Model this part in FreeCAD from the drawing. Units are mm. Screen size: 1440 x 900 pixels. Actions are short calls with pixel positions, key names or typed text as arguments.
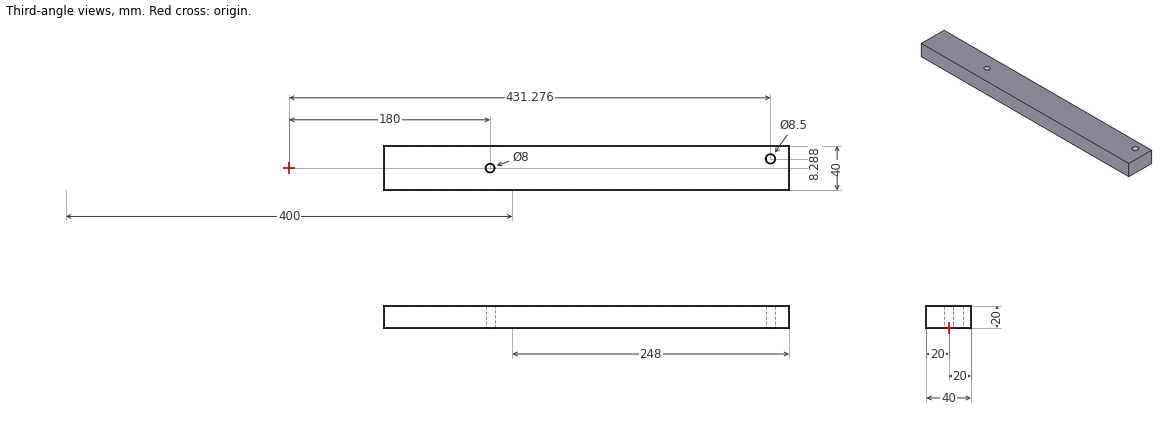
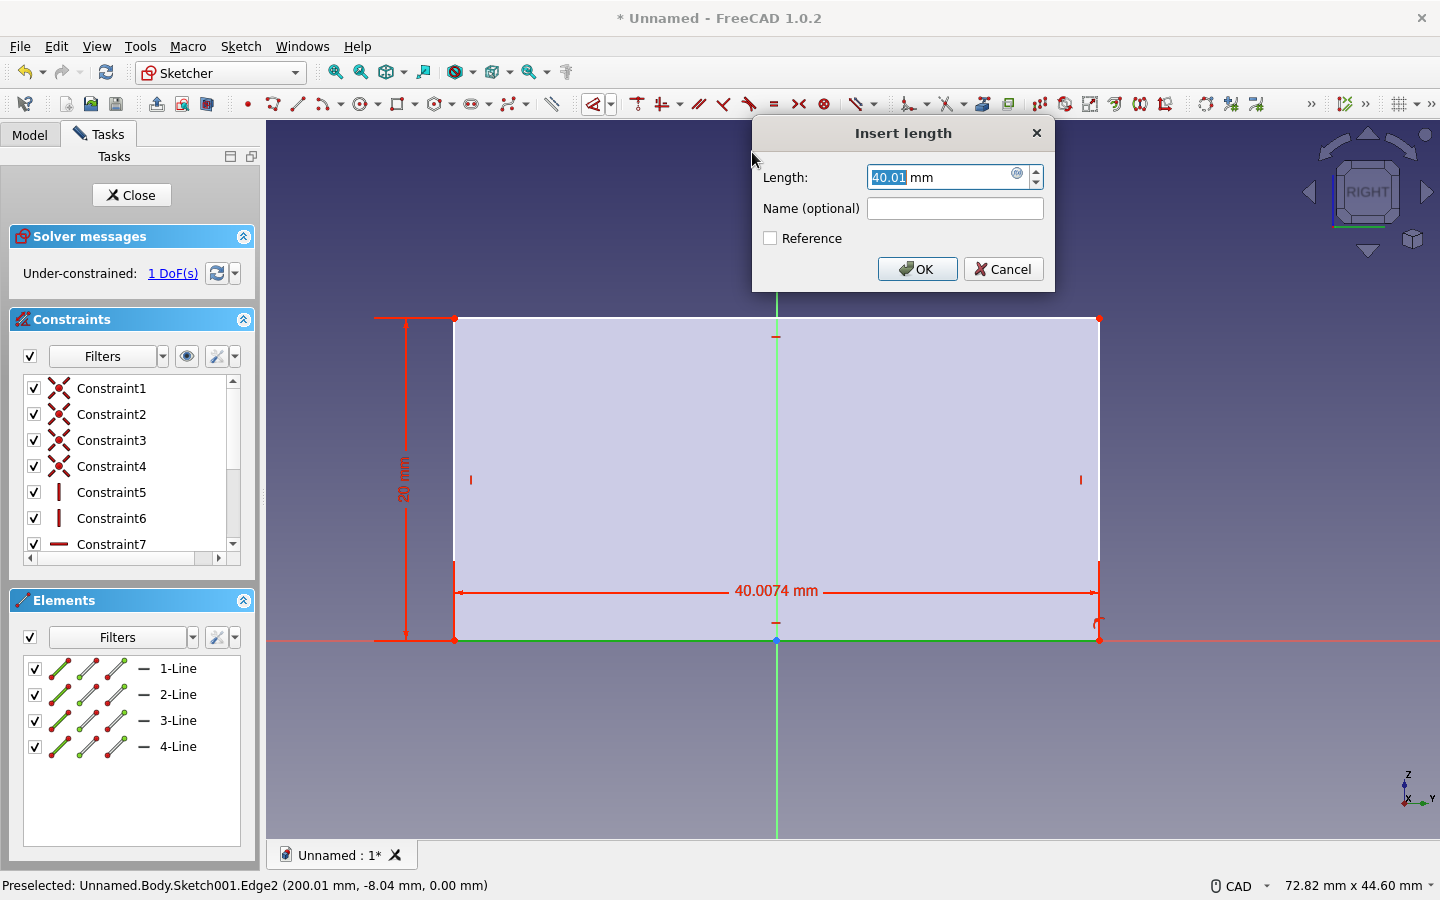
text(40)
key(Return)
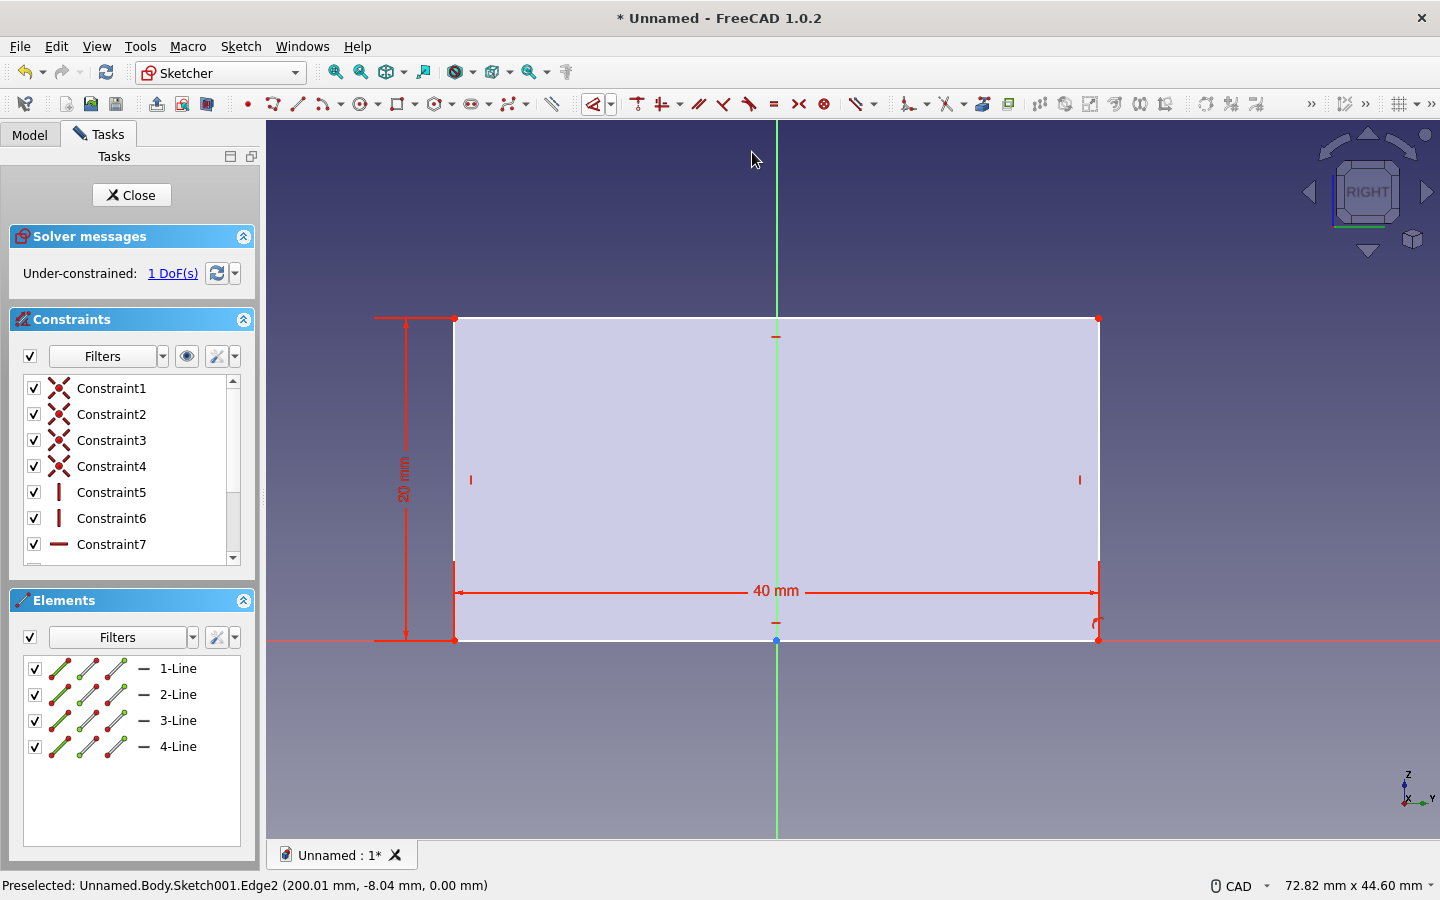
click(454, 318)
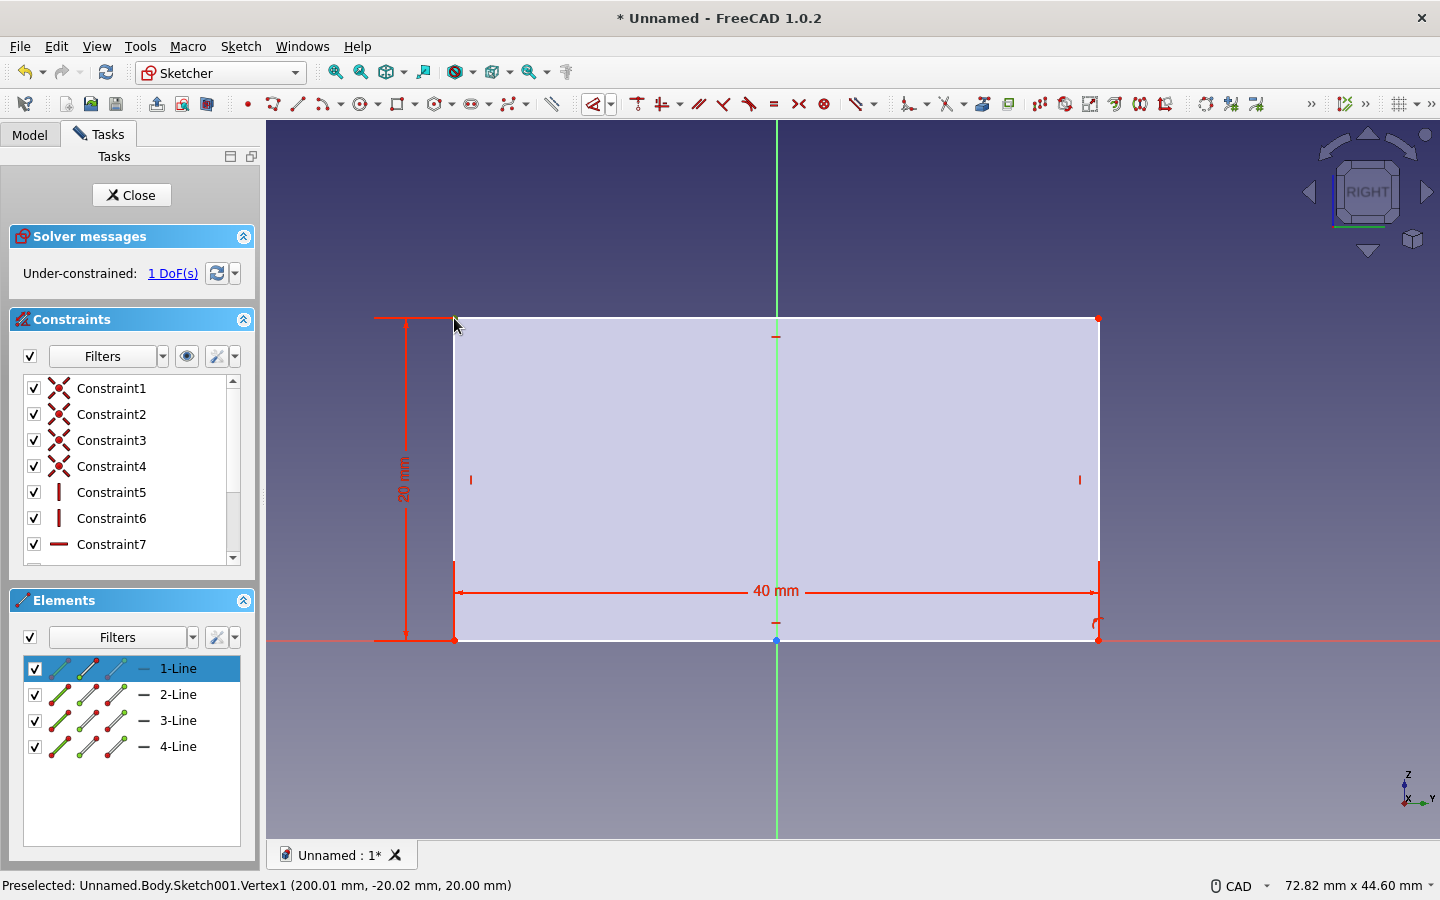
click(610, 104)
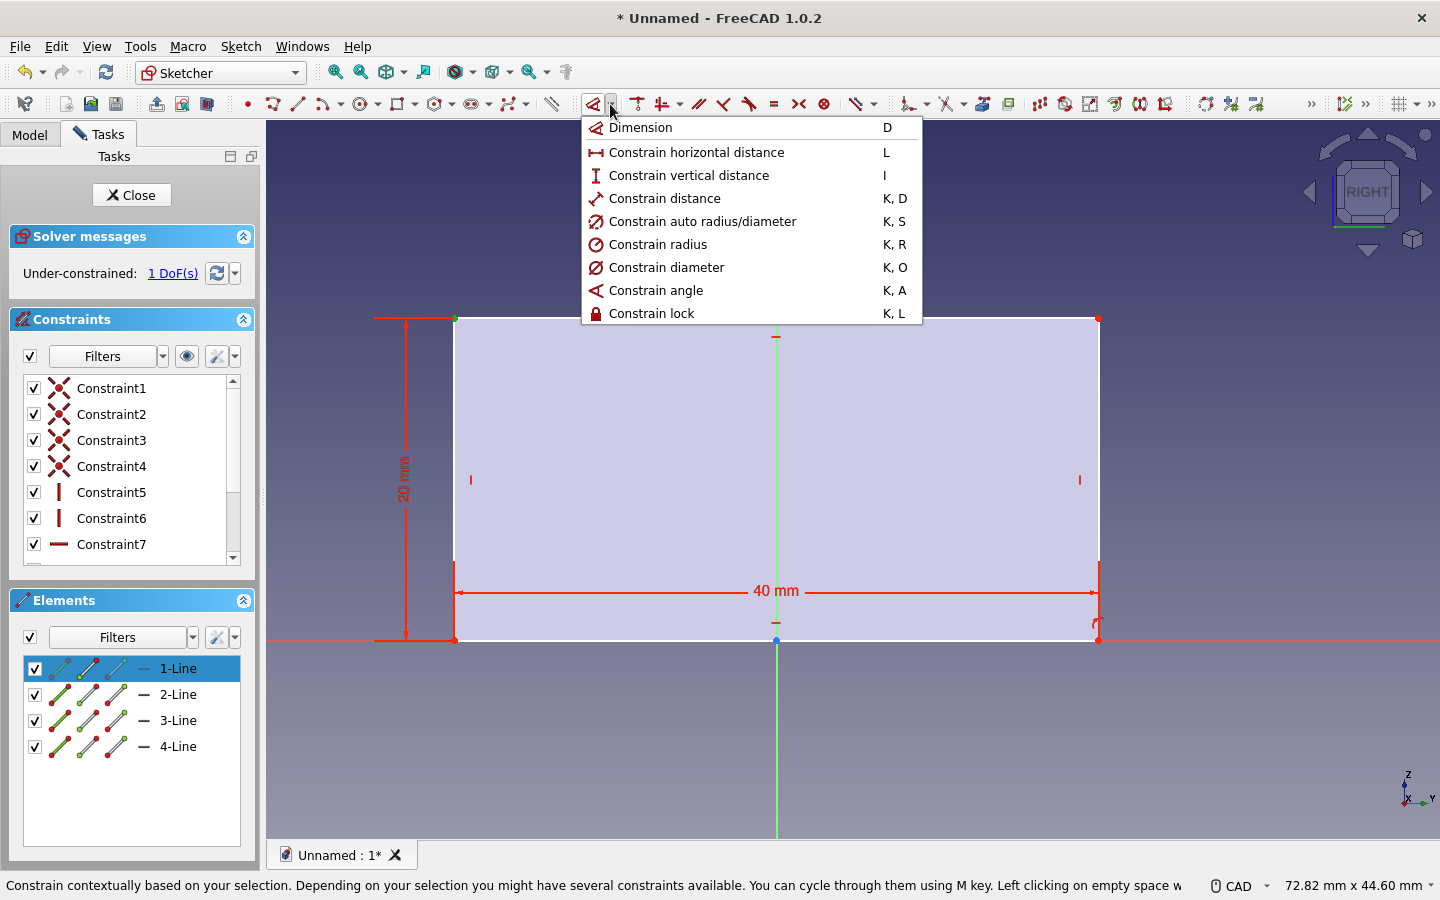
click(752, 152)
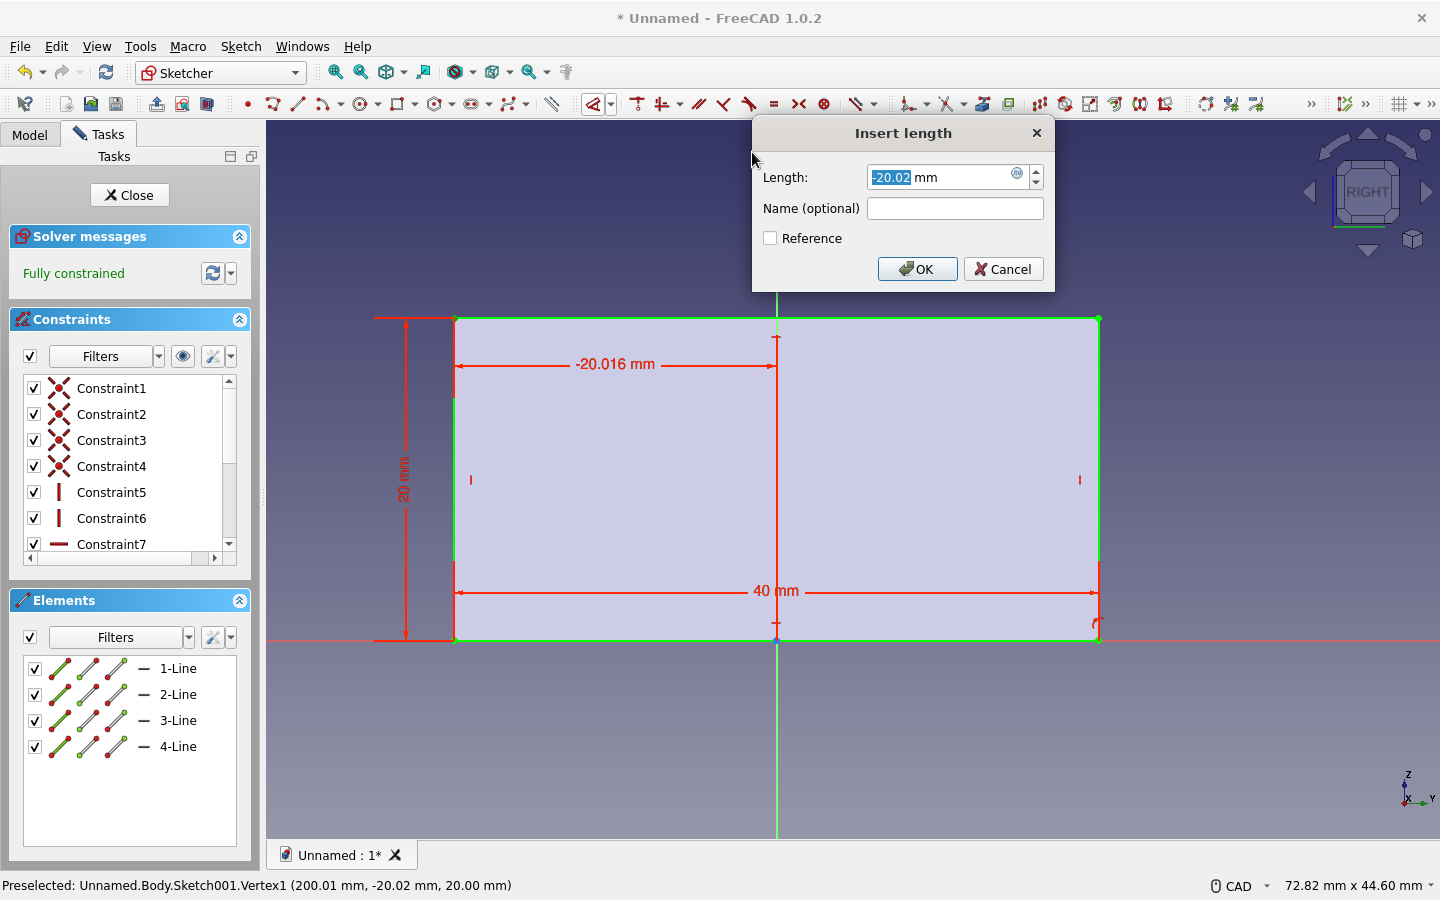
text(-20)
key(Return)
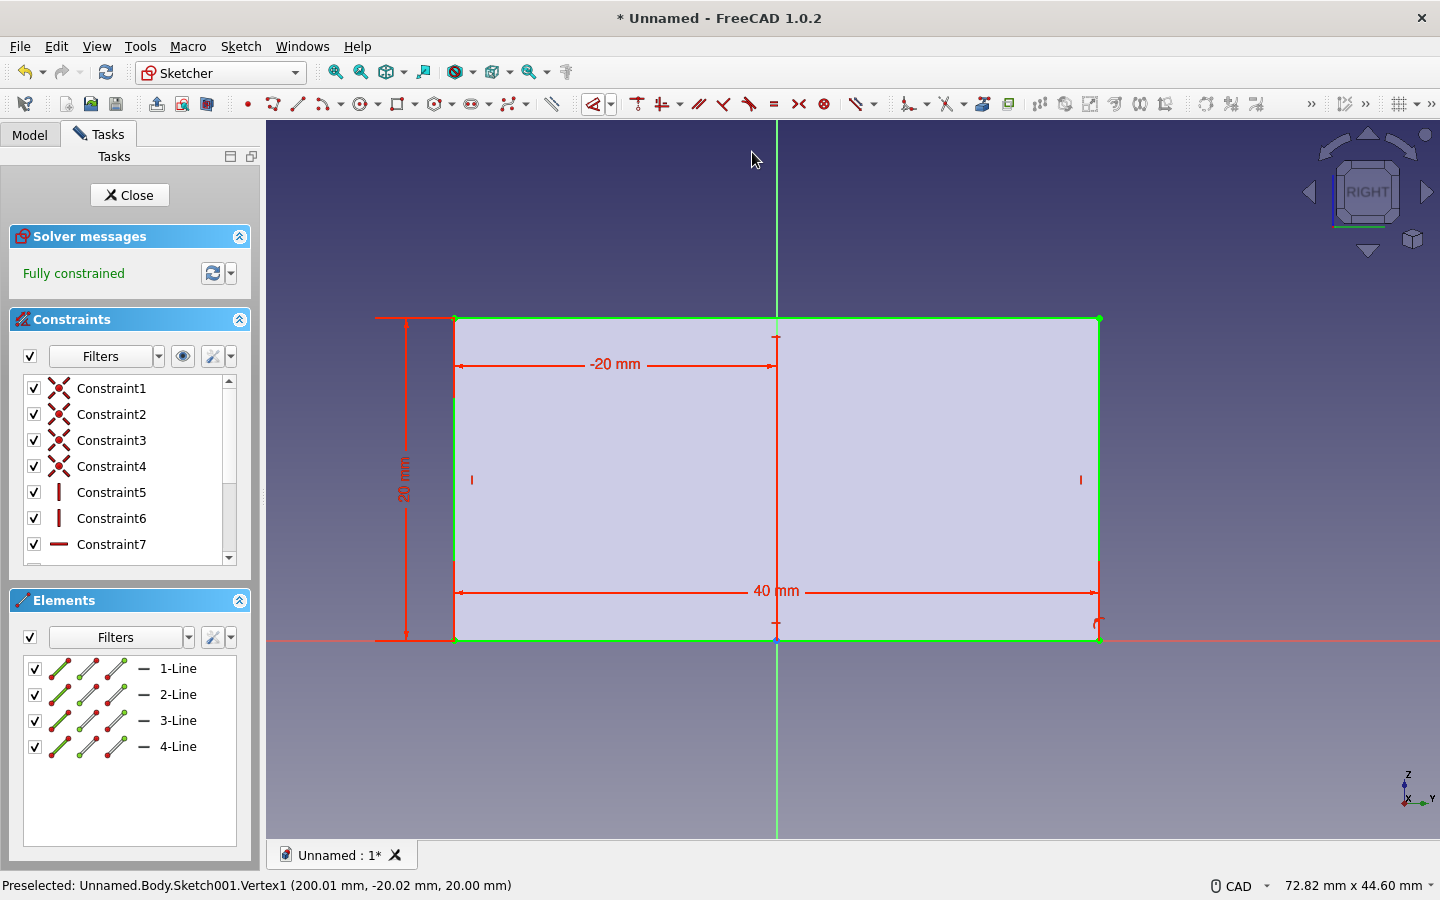
click(130, 195)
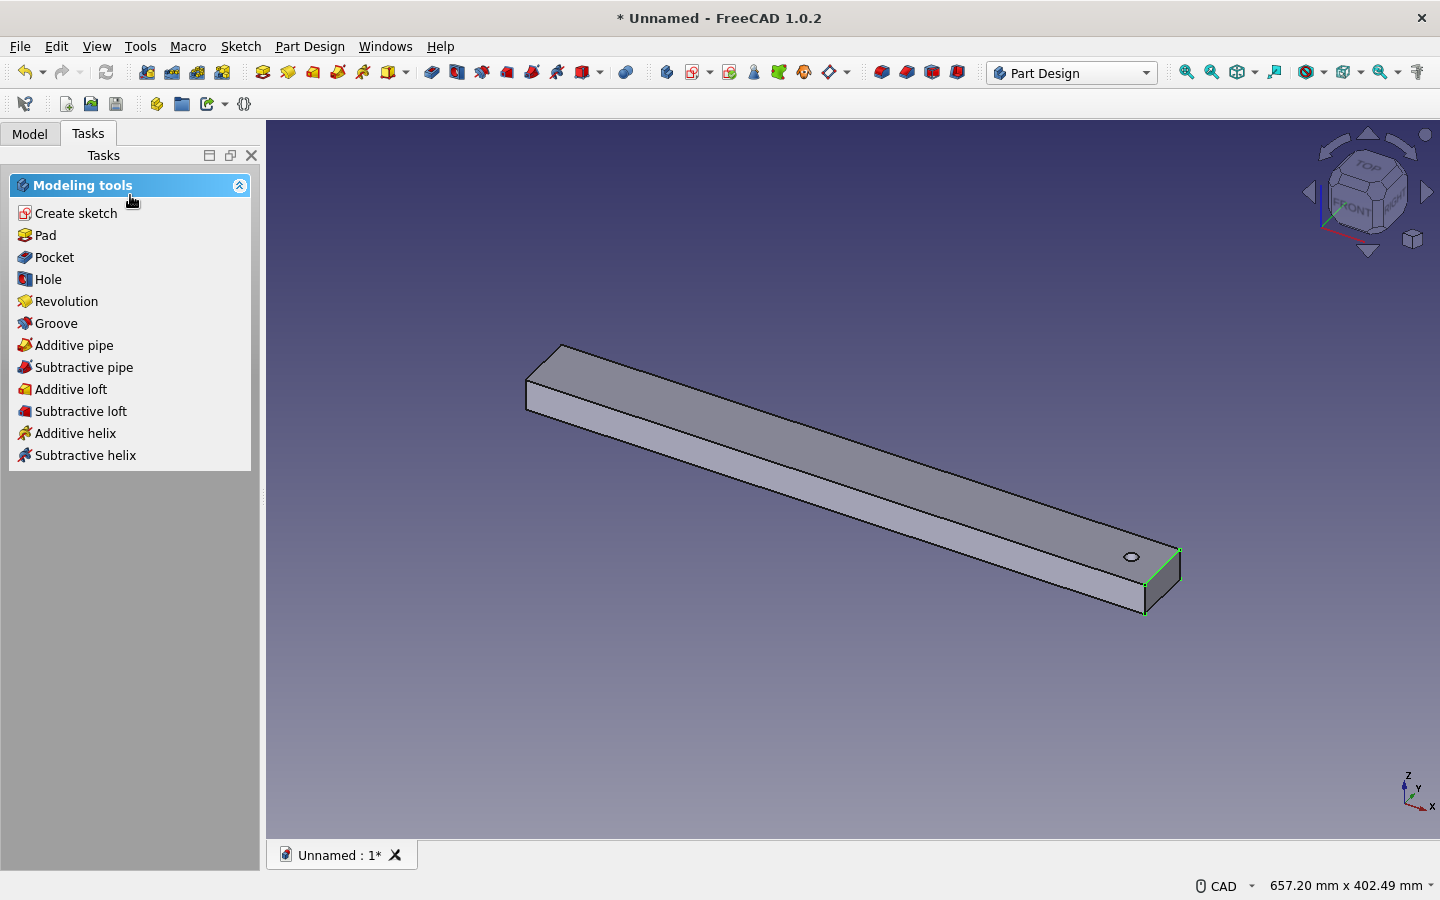
click(263, 72)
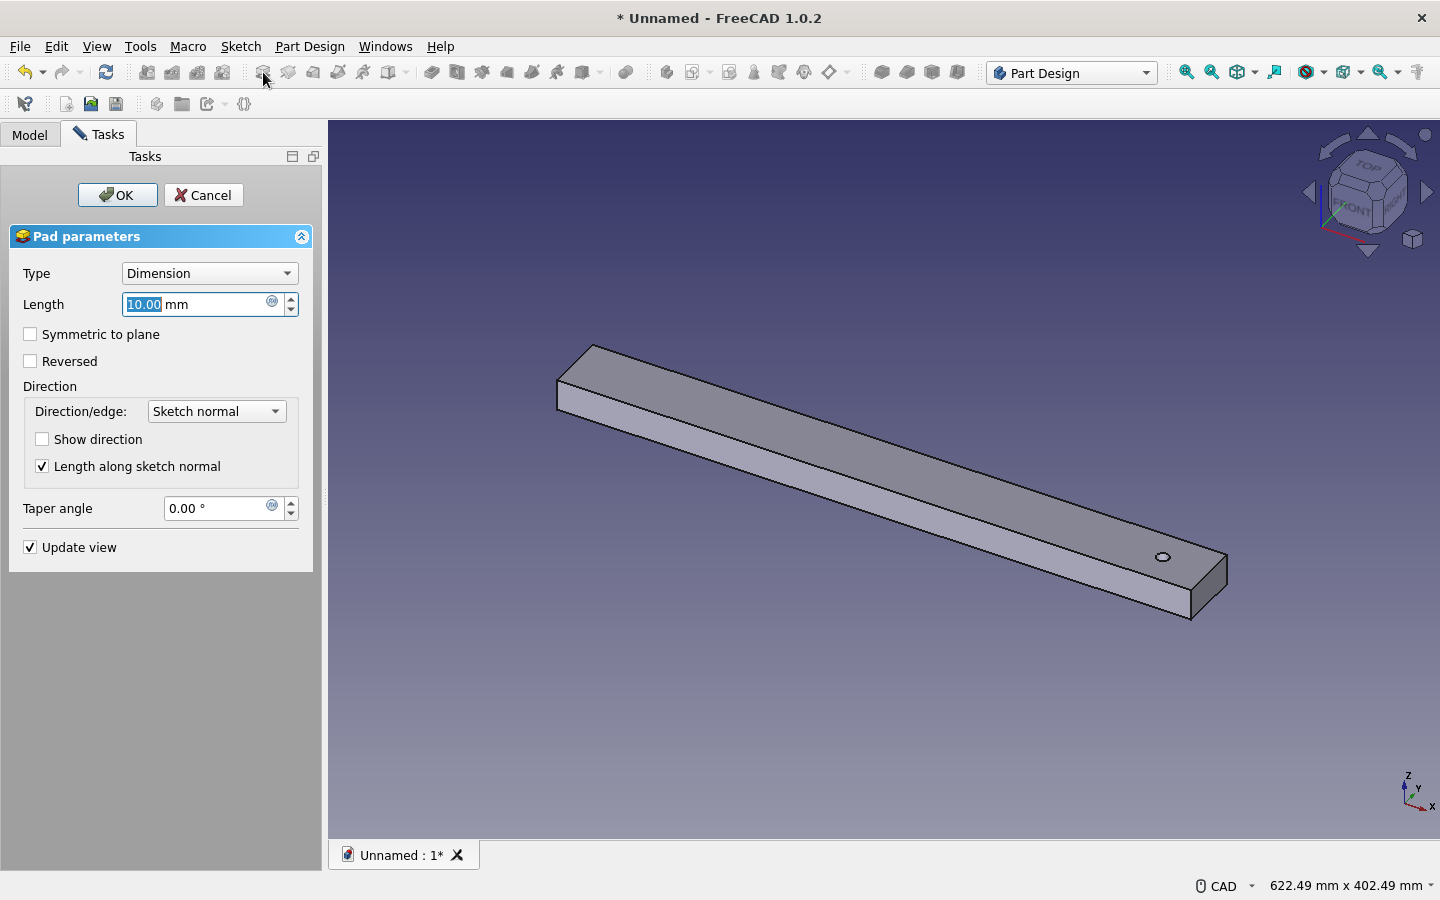
text(248)
key(Tab)